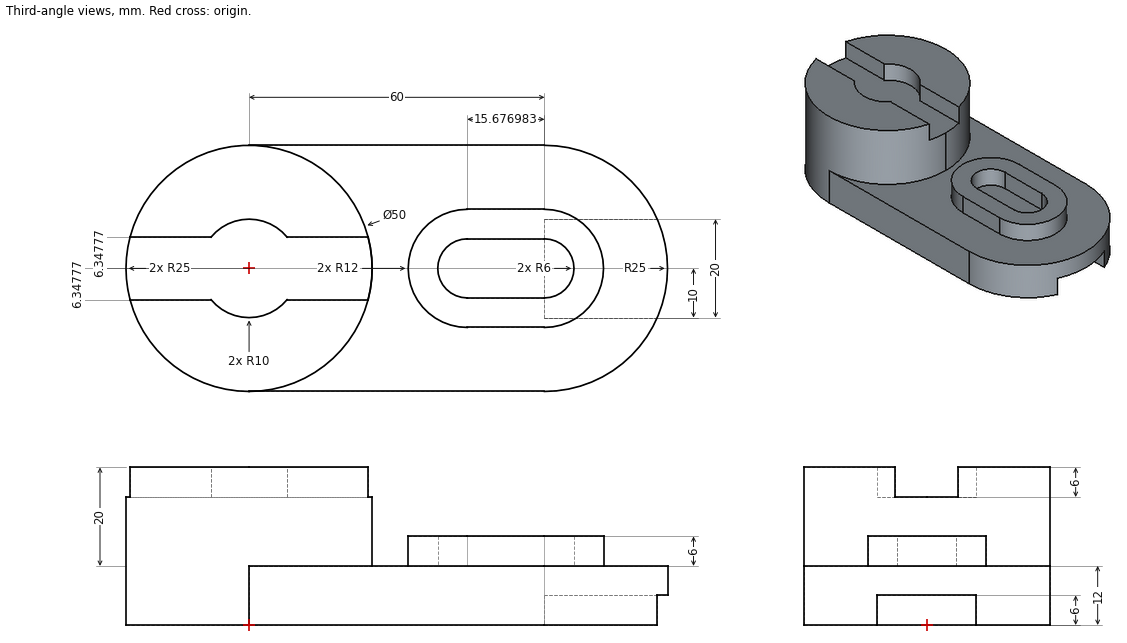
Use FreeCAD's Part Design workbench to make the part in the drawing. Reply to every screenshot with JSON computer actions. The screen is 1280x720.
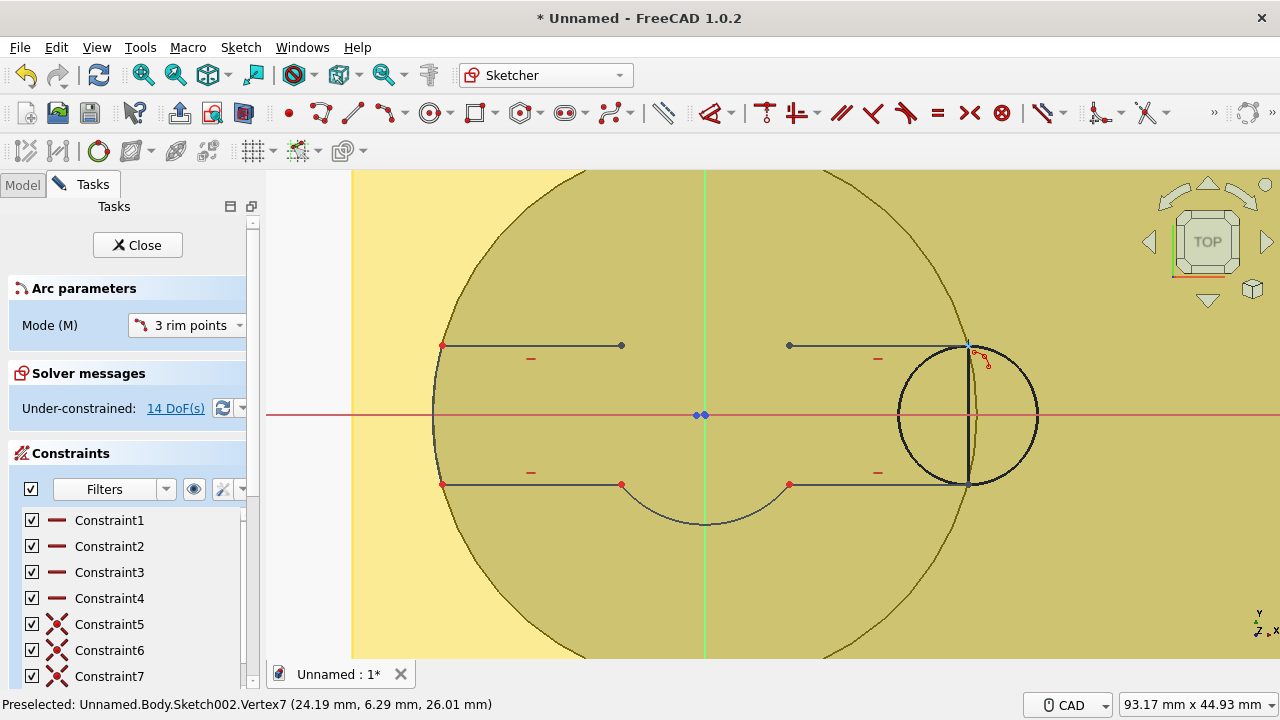
{"action": "scroll", "coordinate": [977, 428], "scroll_direction": "up", "scroll_amount": 4}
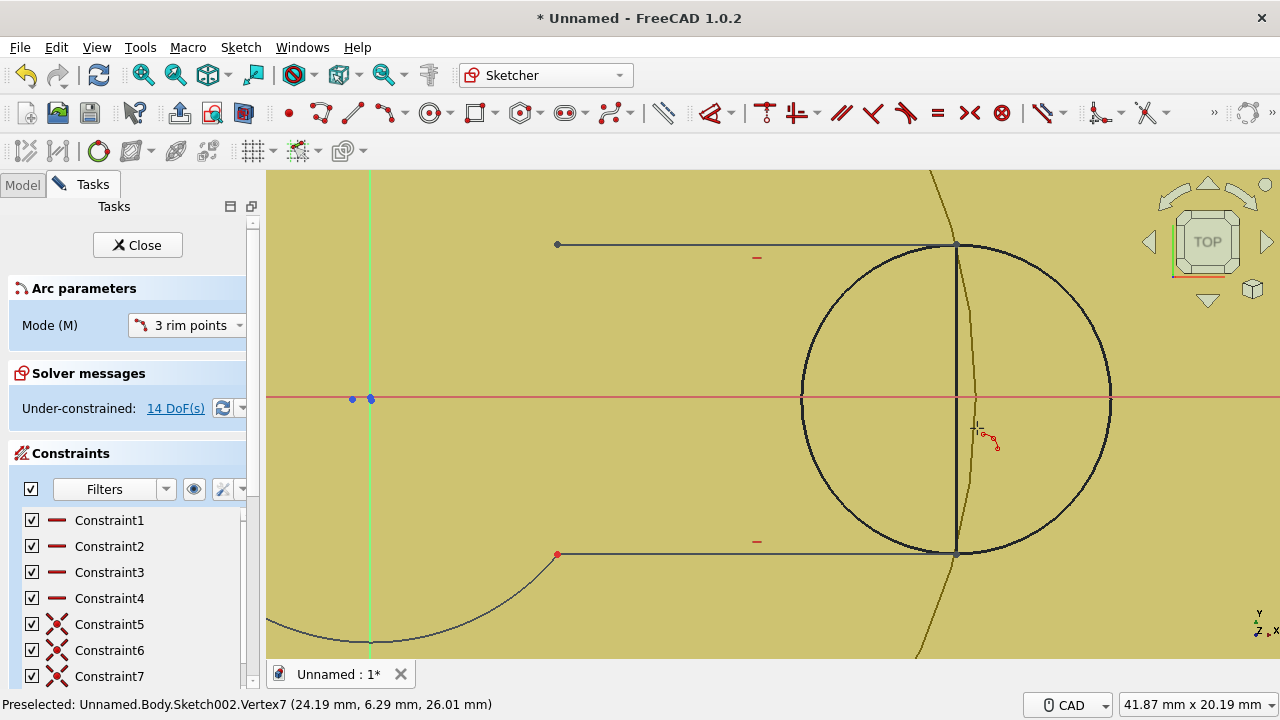
{"action": "left_click", "coordinate": [975, 428]}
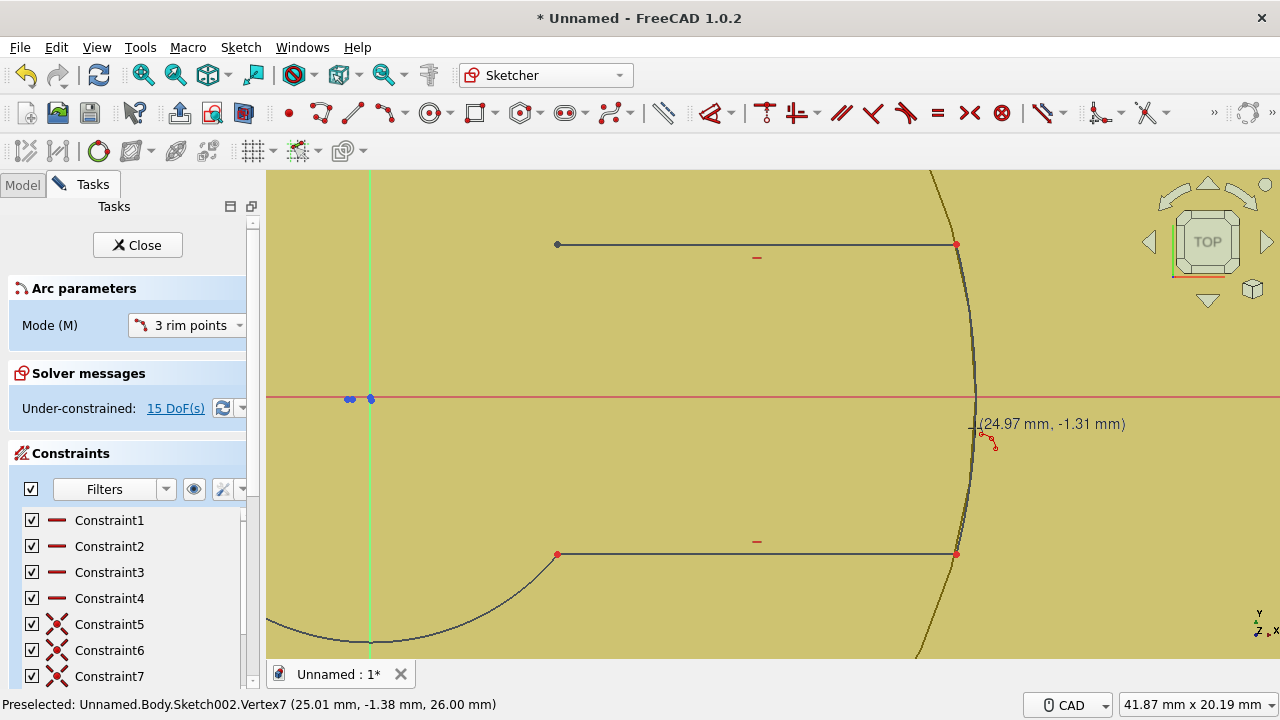
{"action": "left_click", "coordinate": [558, 245]}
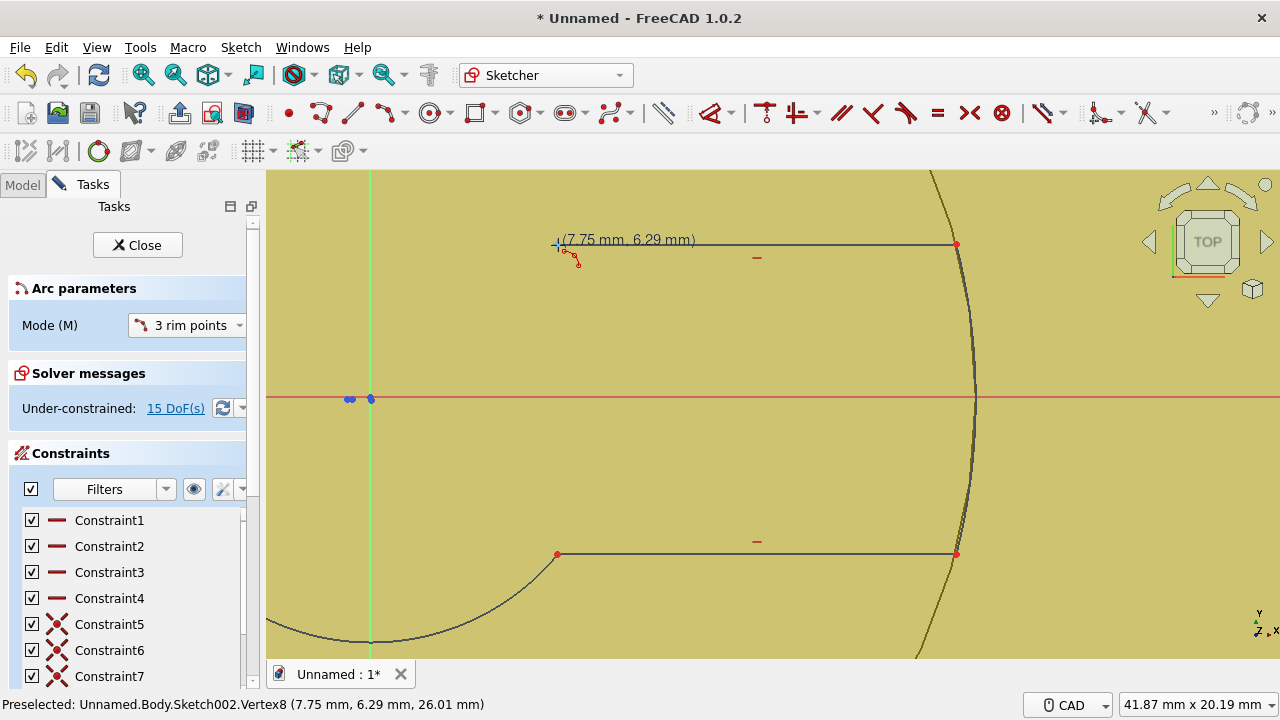
{"action": "scroll", "coordinate": [977, 429], "scroll_direction": "down", "scroll_amount": 4}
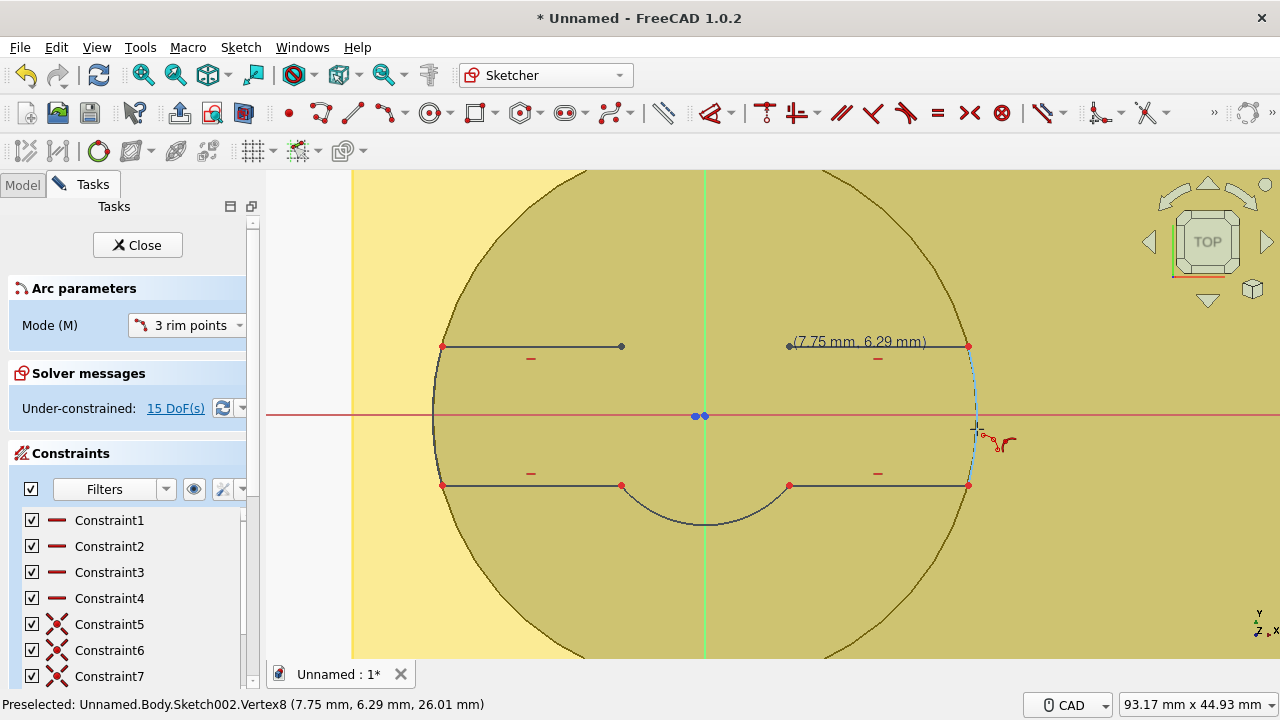
{"action": "left_click", "coordinate": [621, 347]}
{"action": "left_click", "coordinate": [724, 308]}
{"action": "key", "text": "Escape"}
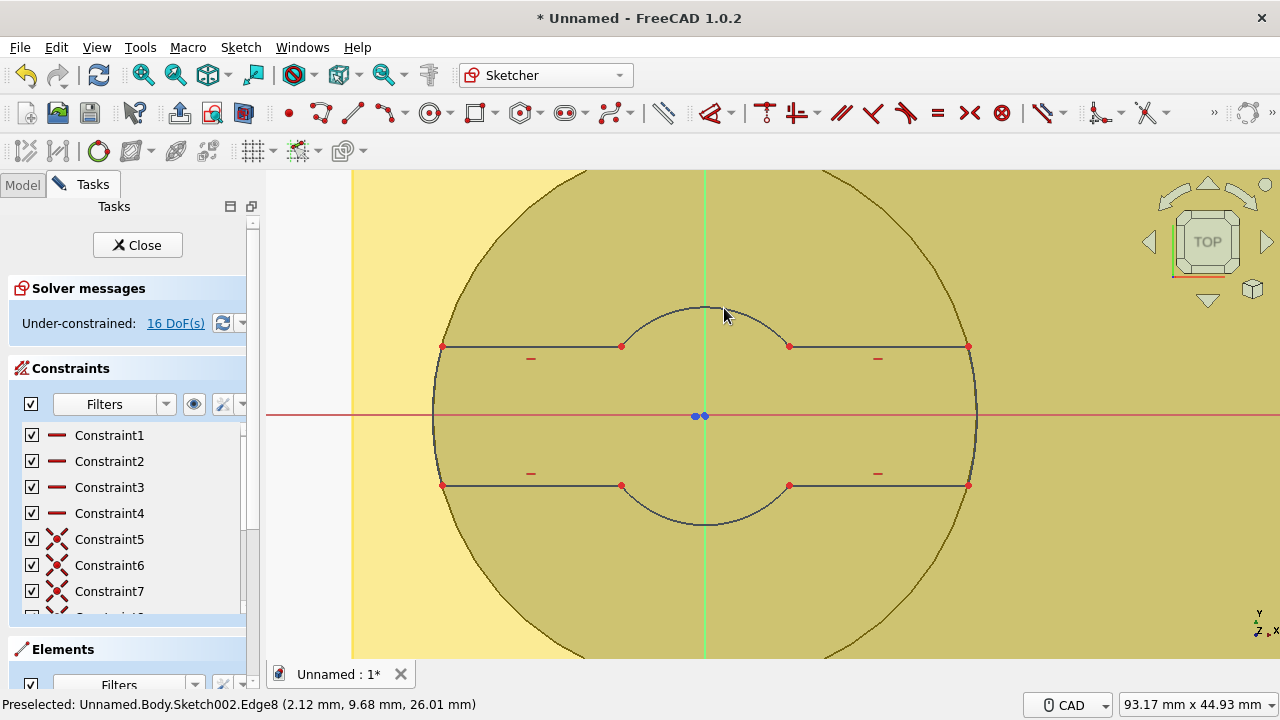
{"action": "left_click", "coordinate": [434, 388]}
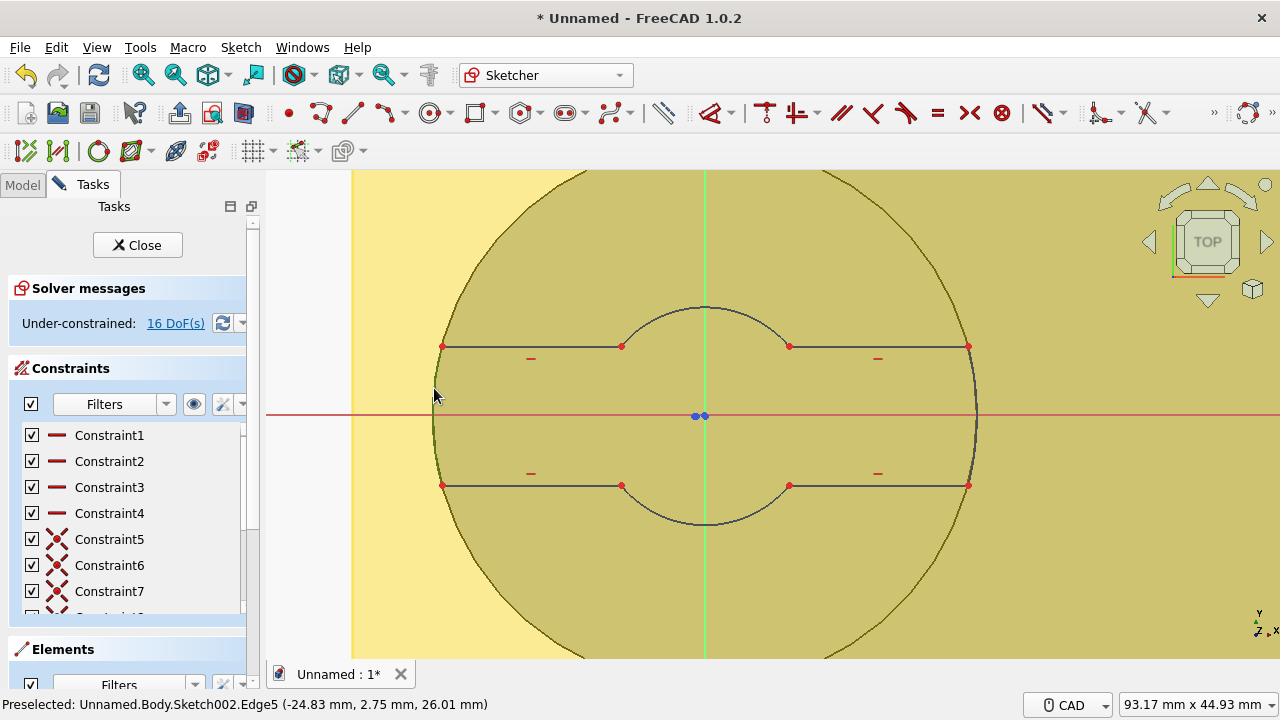
{"action": "left_click", "coordinate": [667, 519]}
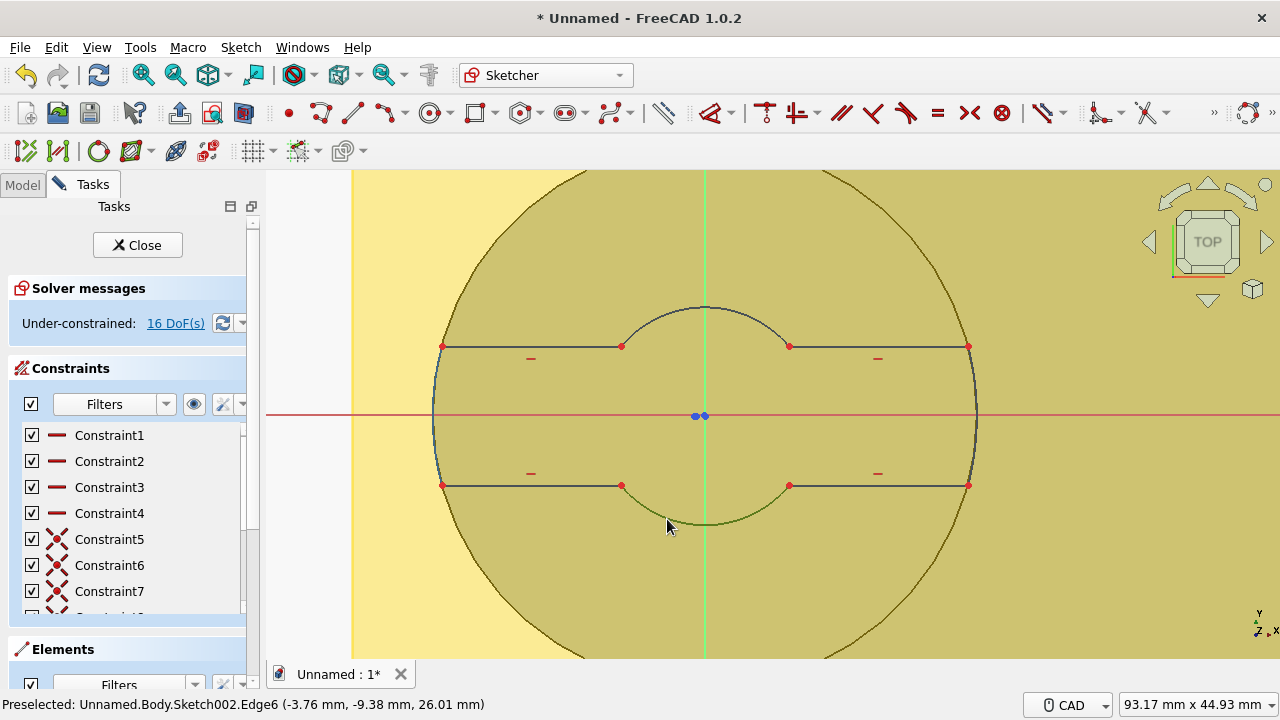
{"action": "key", "text": "c"}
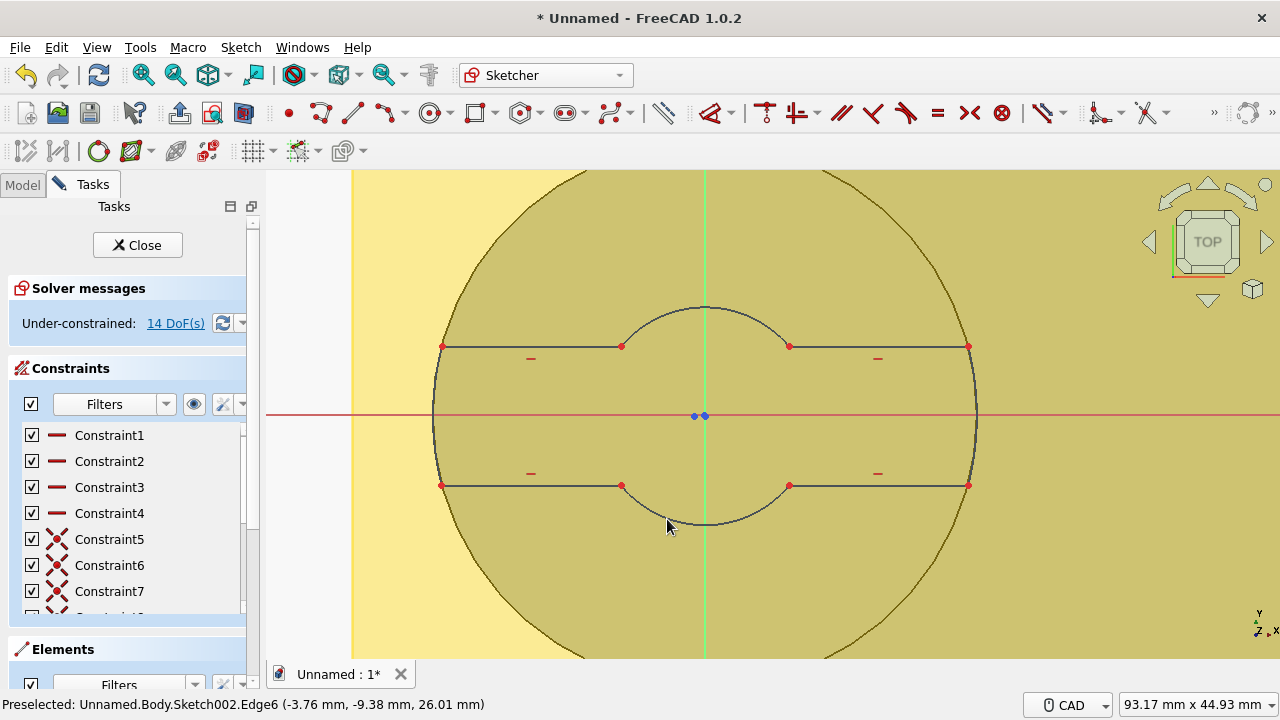
{"action": "left_click", "coordinate": [435, 388]}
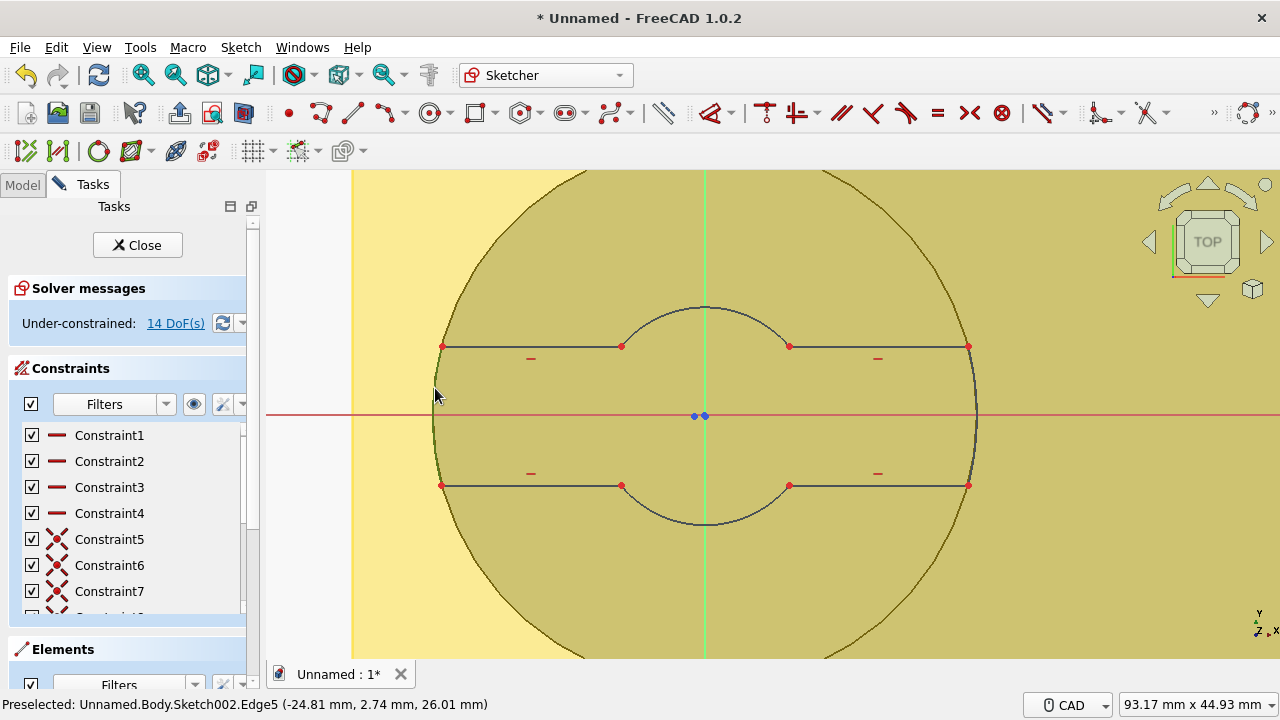
{"action": "left_click", "coordinate": [975, 444]}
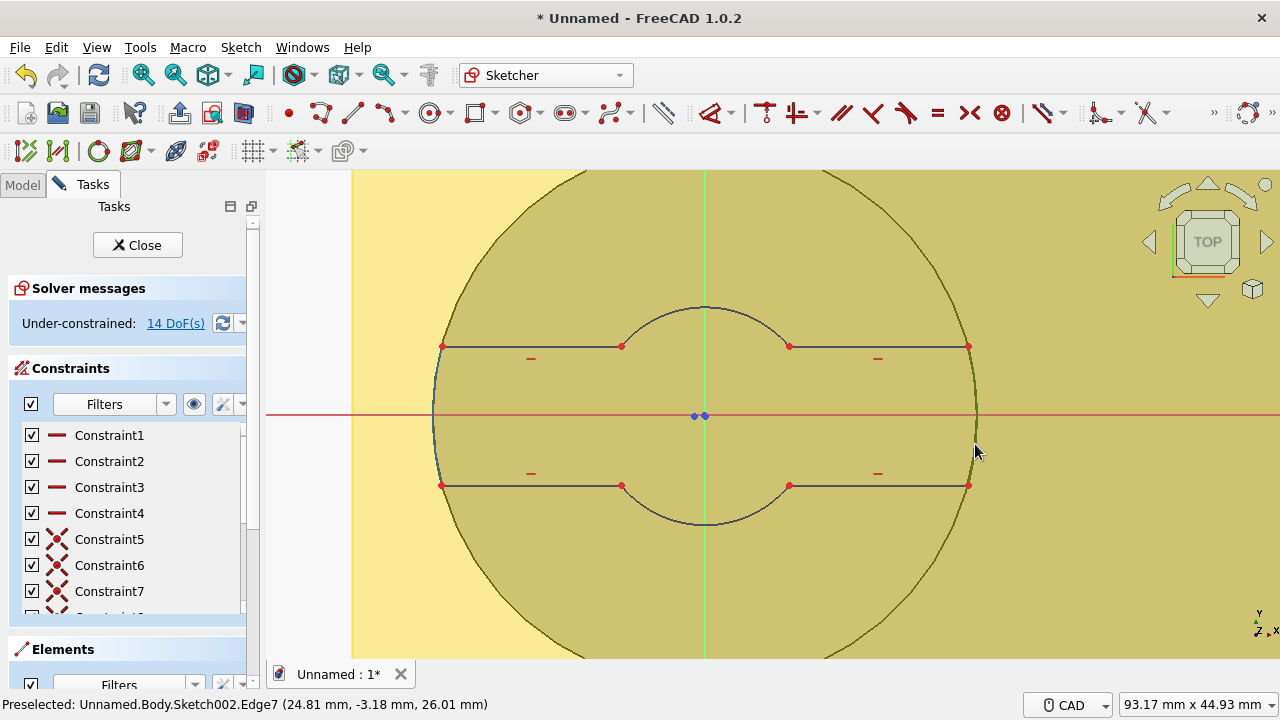
{"action": "key", "text": "c"}